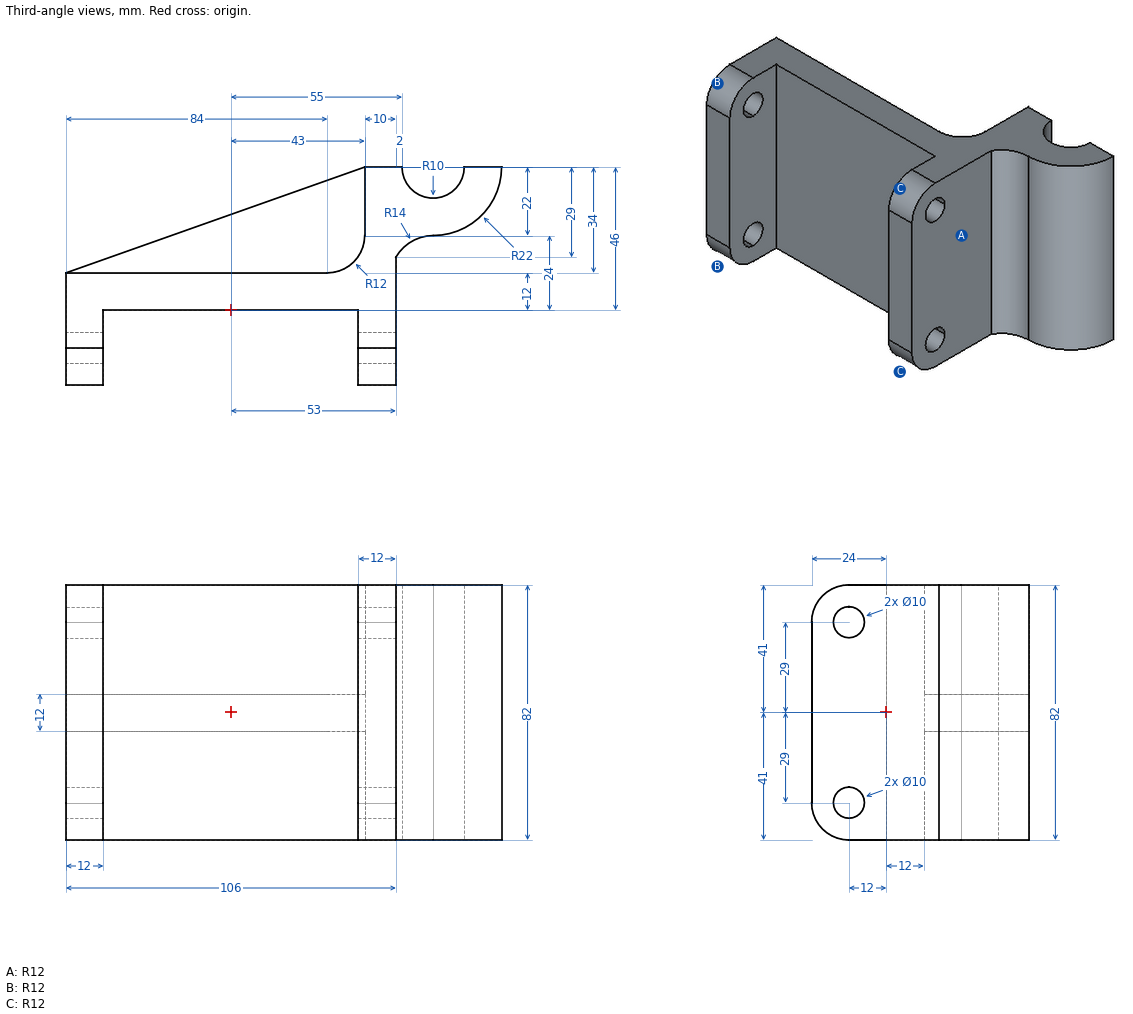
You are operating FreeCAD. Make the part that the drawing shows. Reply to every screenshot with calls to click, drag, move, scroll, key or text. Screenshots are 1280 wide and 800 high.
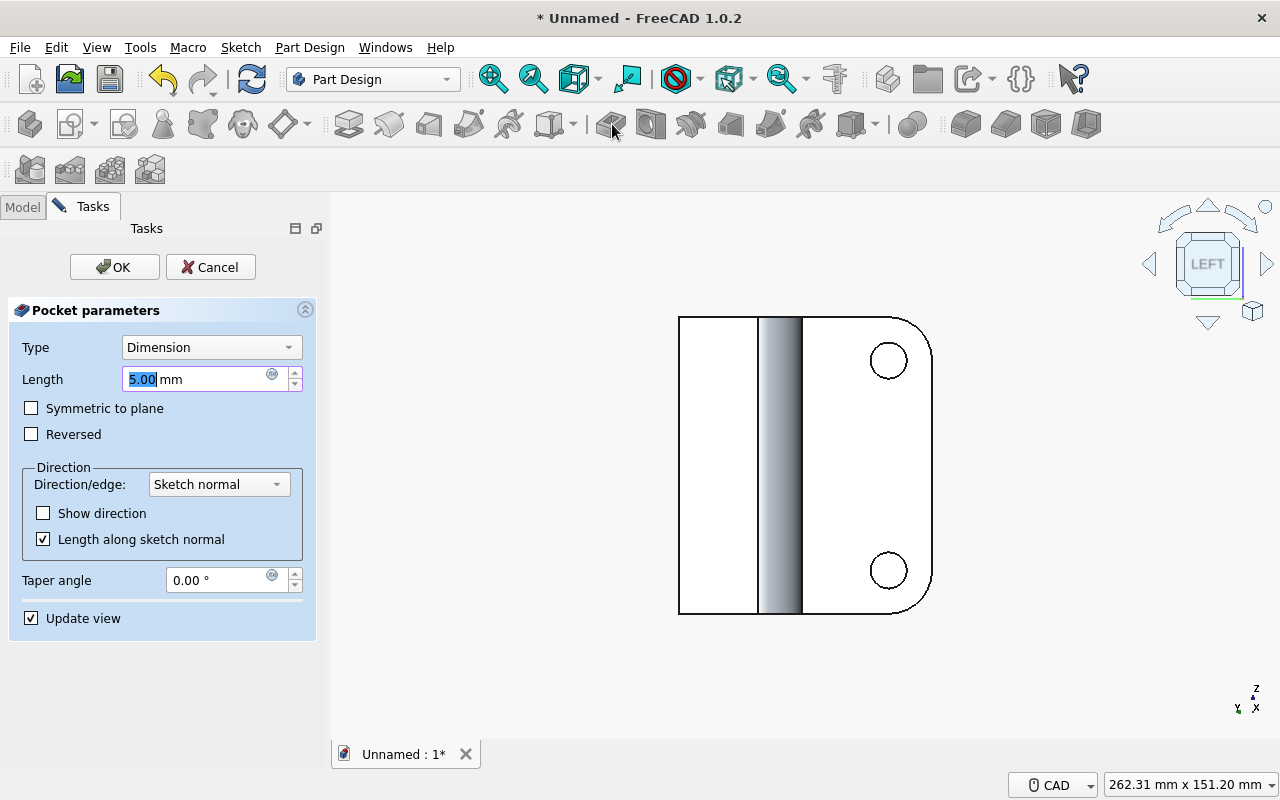
click(212, 348)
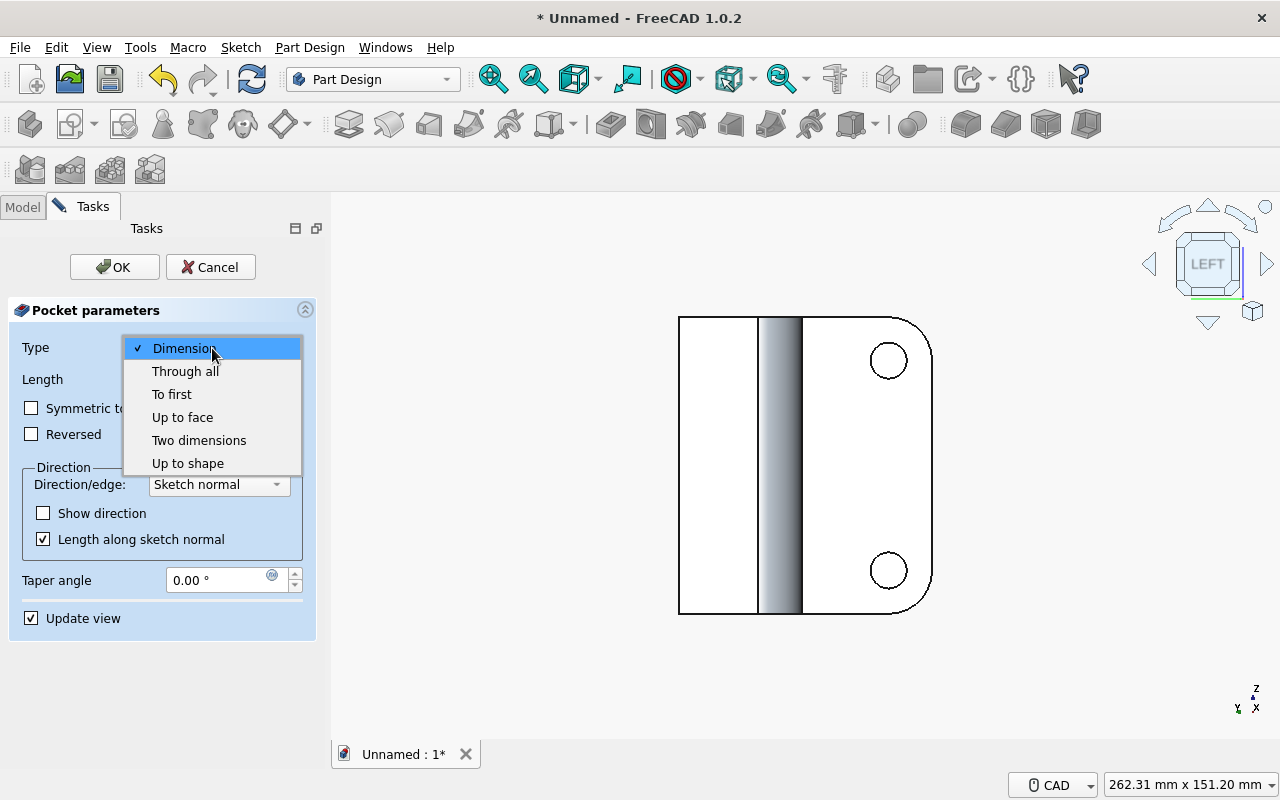
click(212, 372)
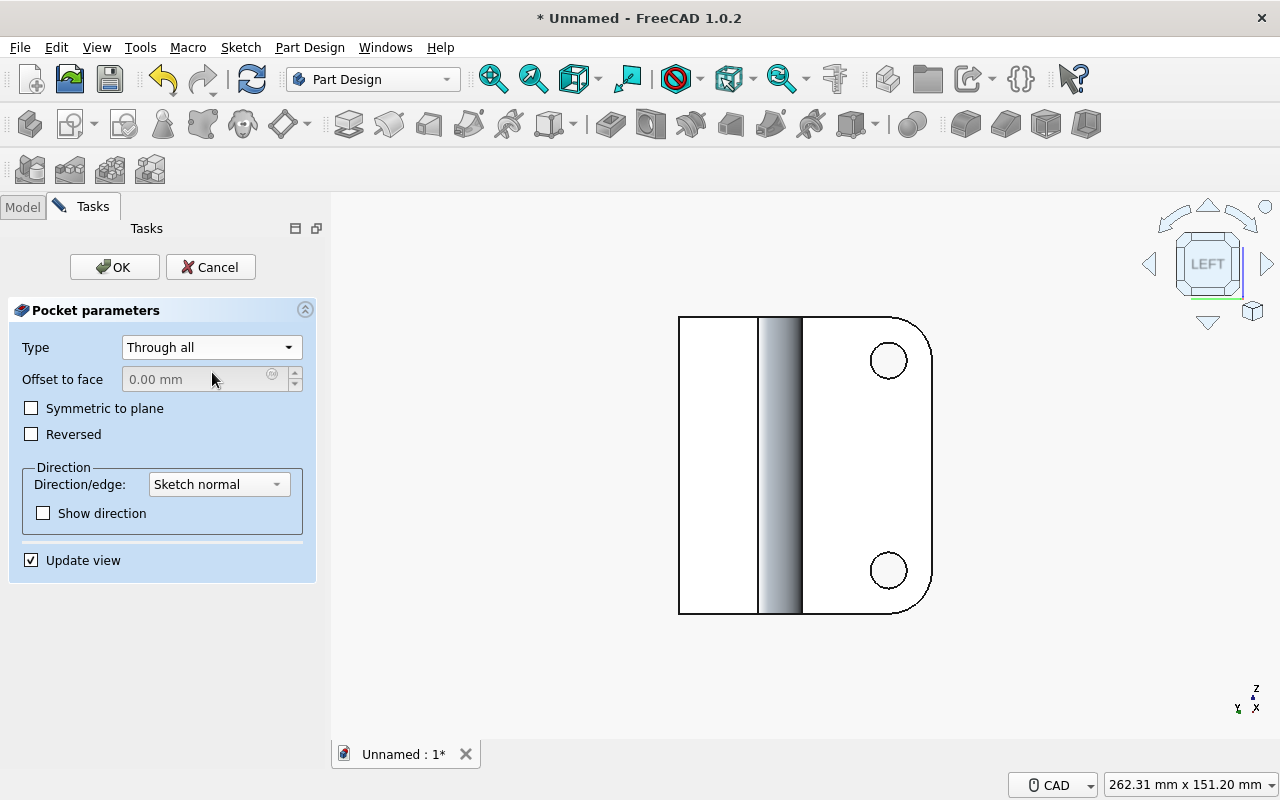
click(115, 267)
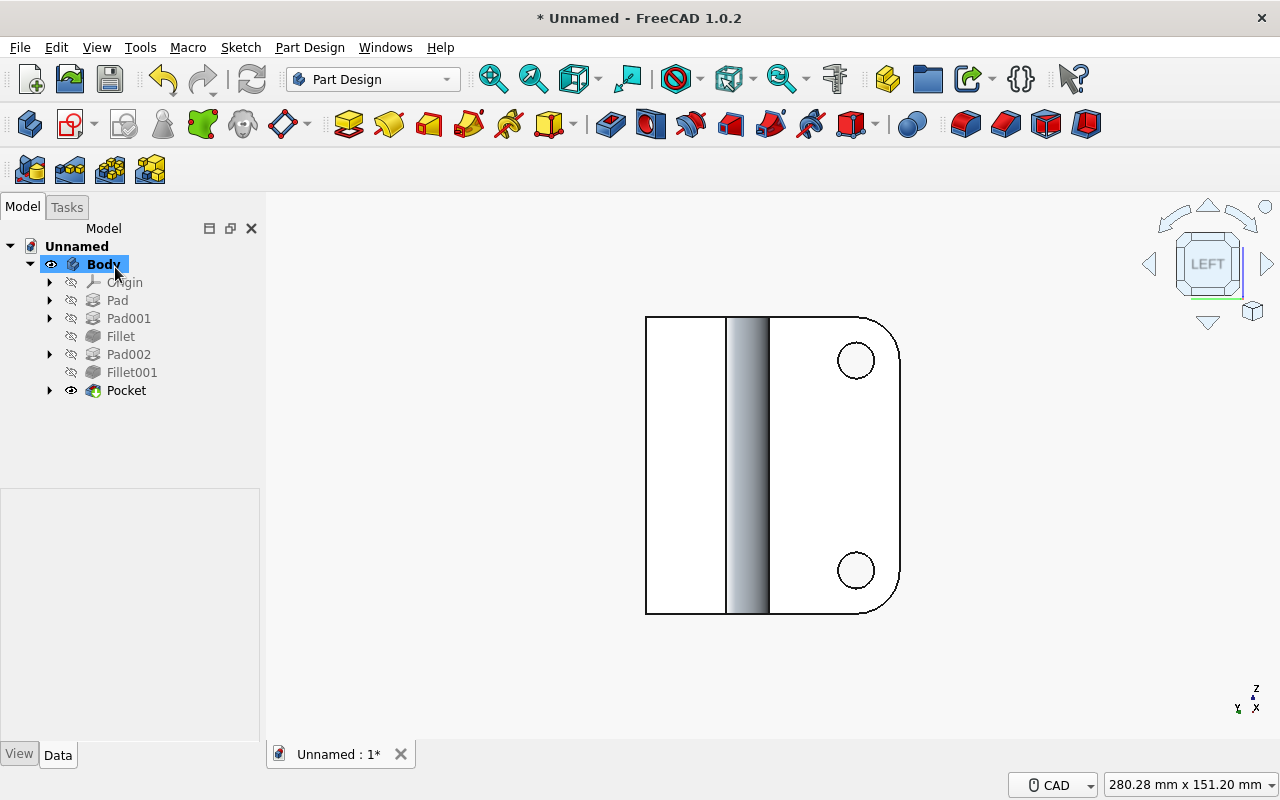
key(0)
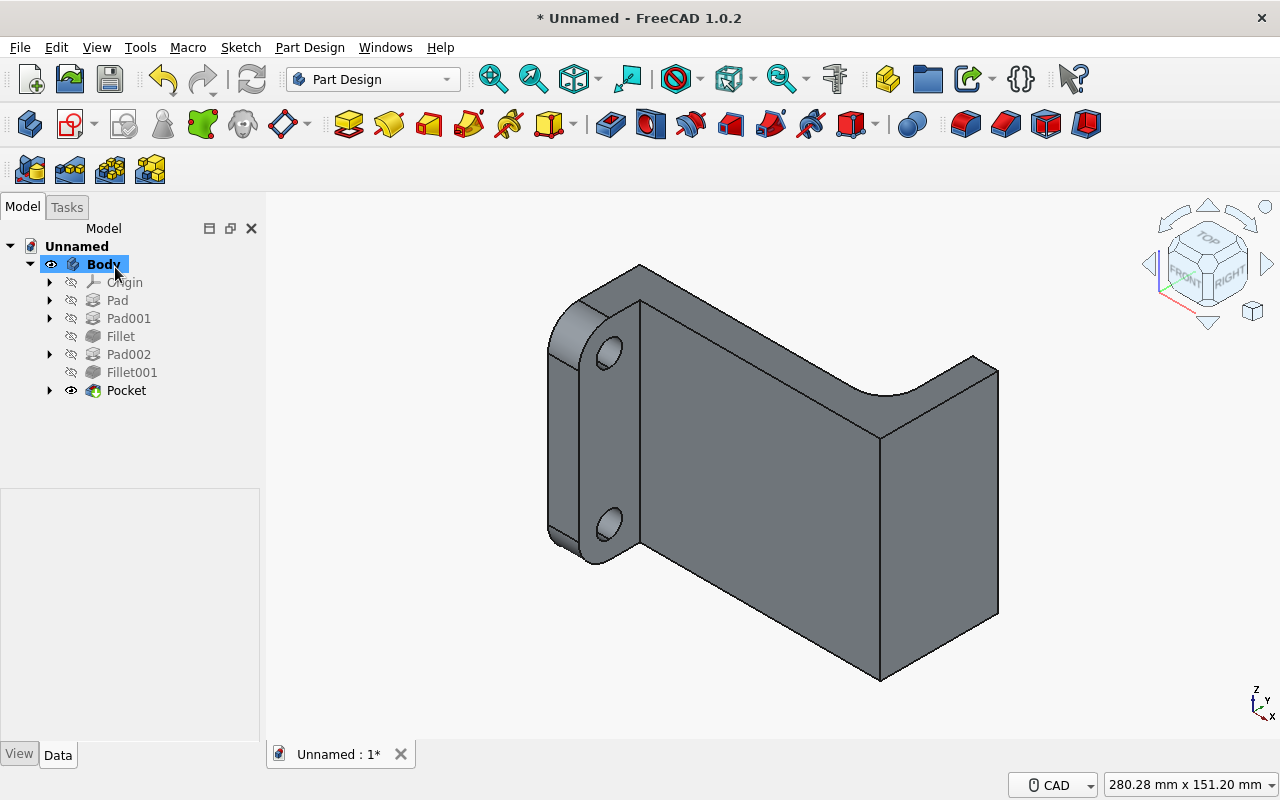
click(939, 560)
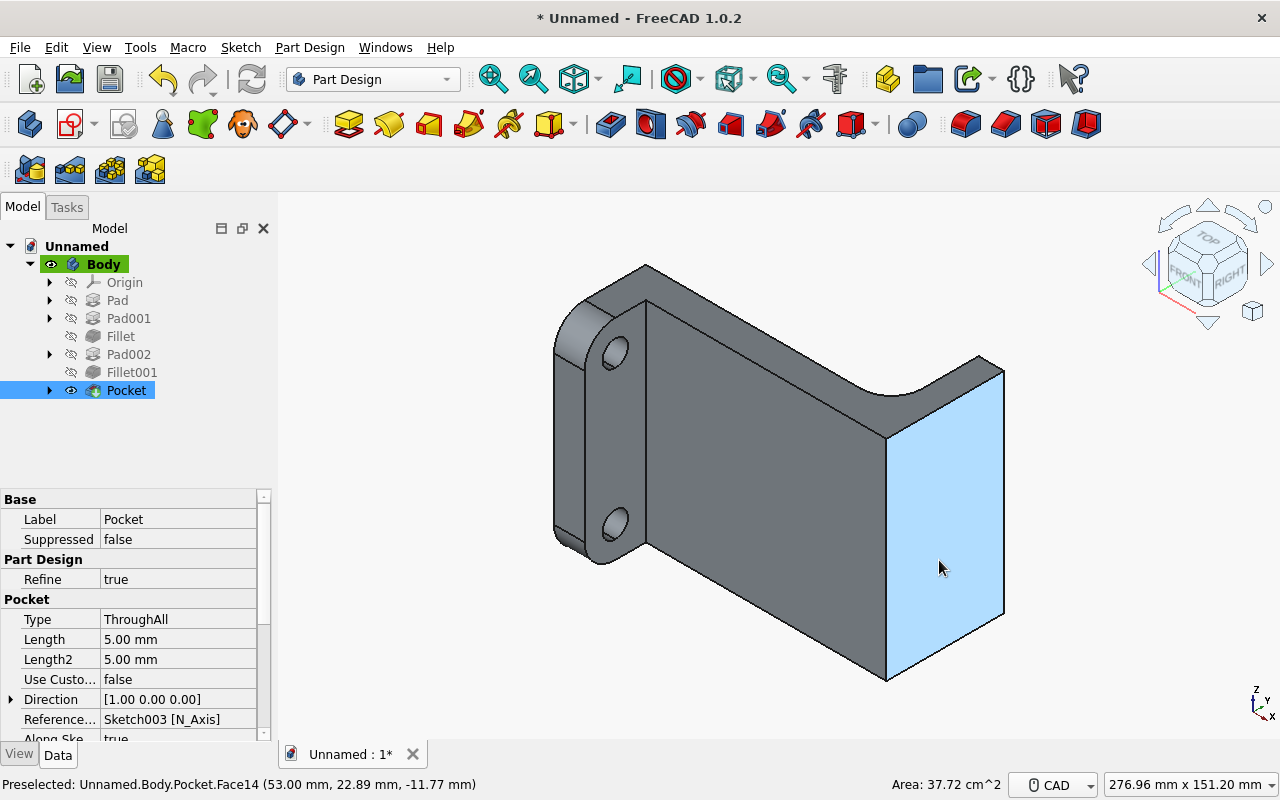
click(70, 124)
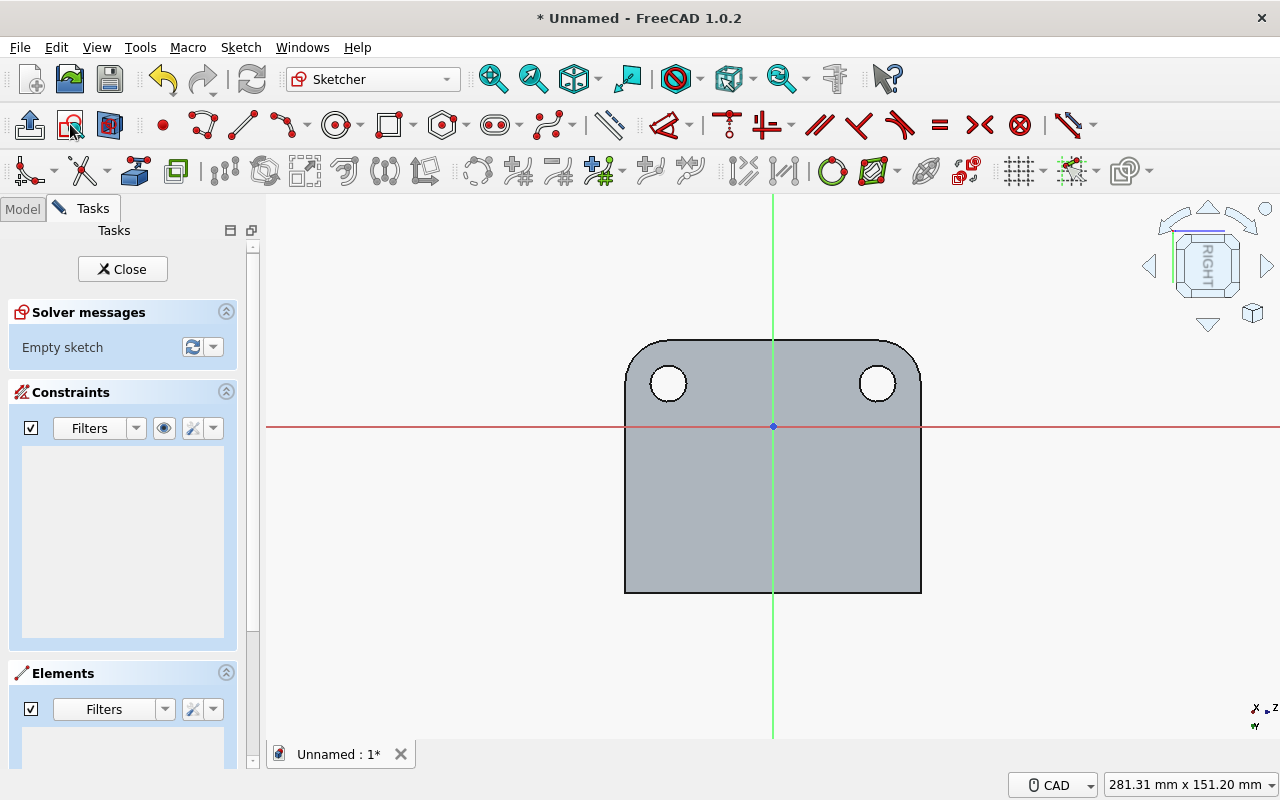
scroll(856, 283, up, 3)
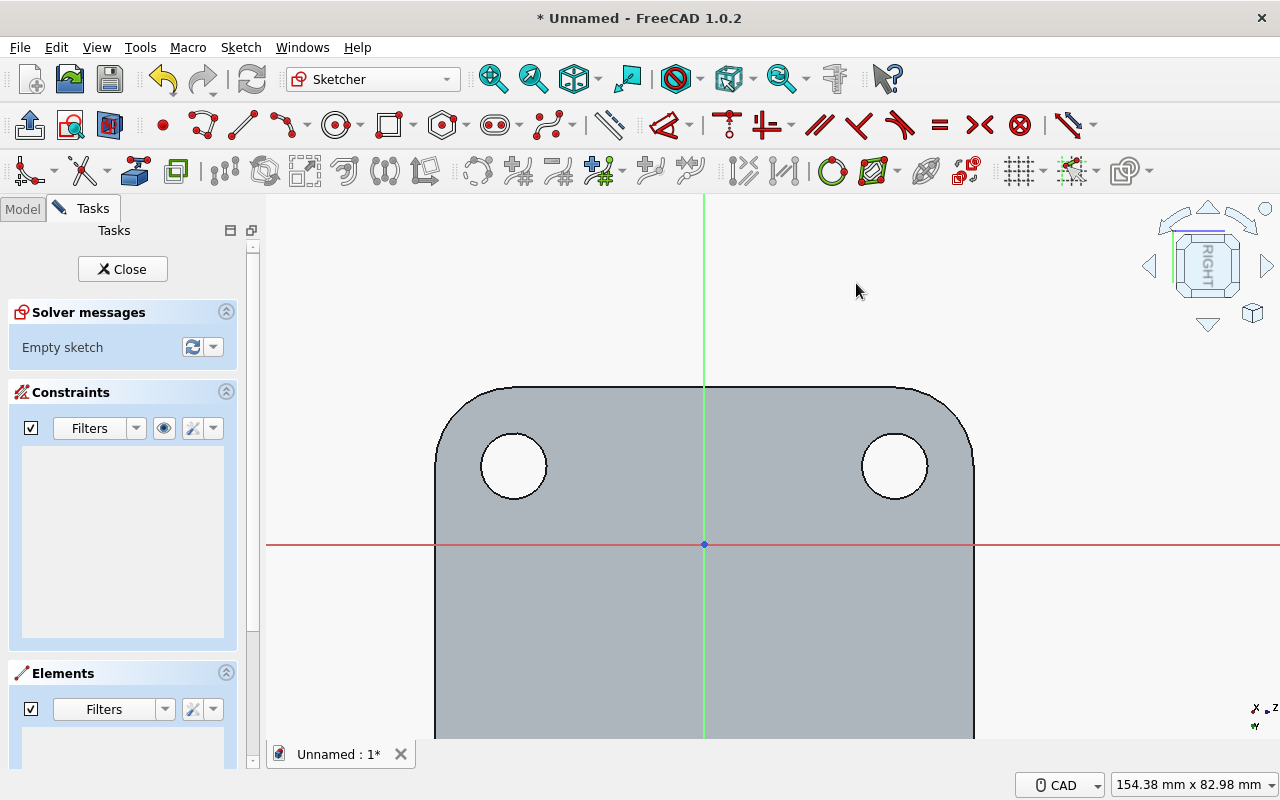
key(g)
key(r)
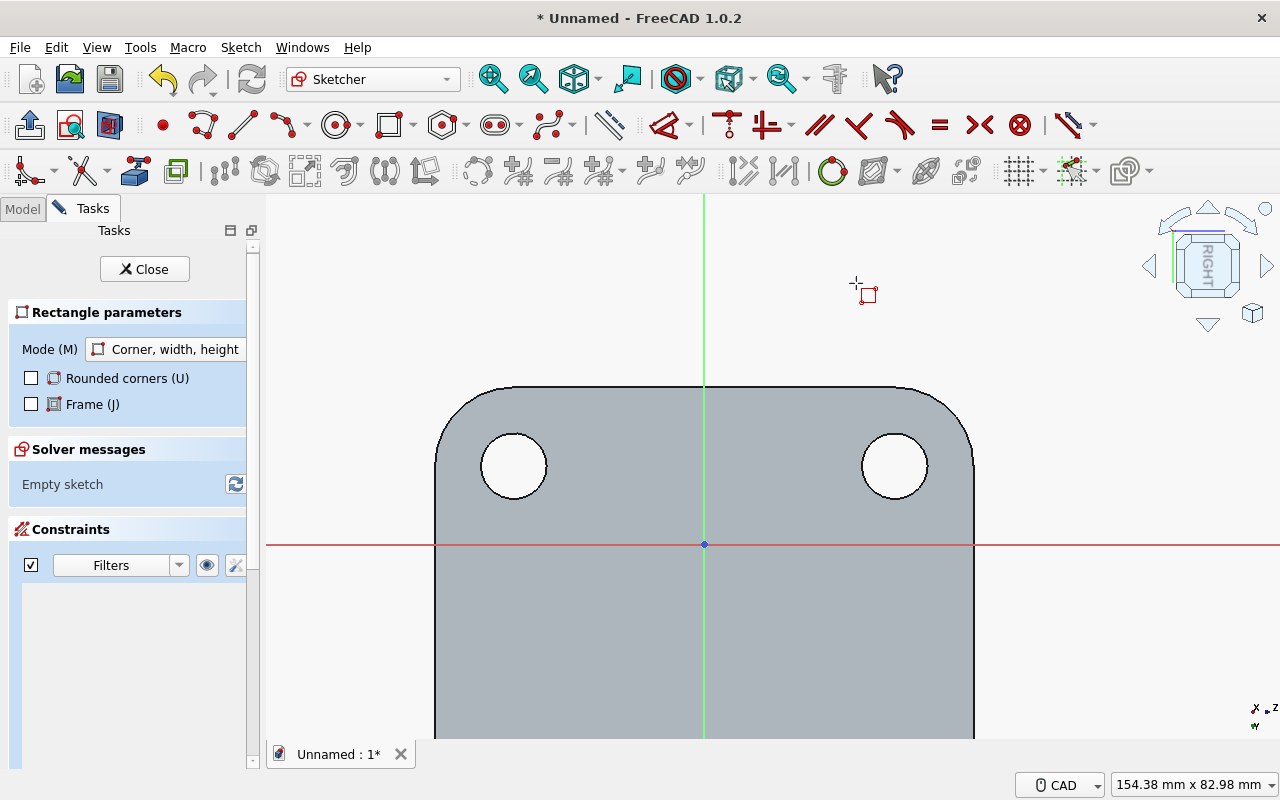
click(435, 387)
click(974, 545)
key(Escape)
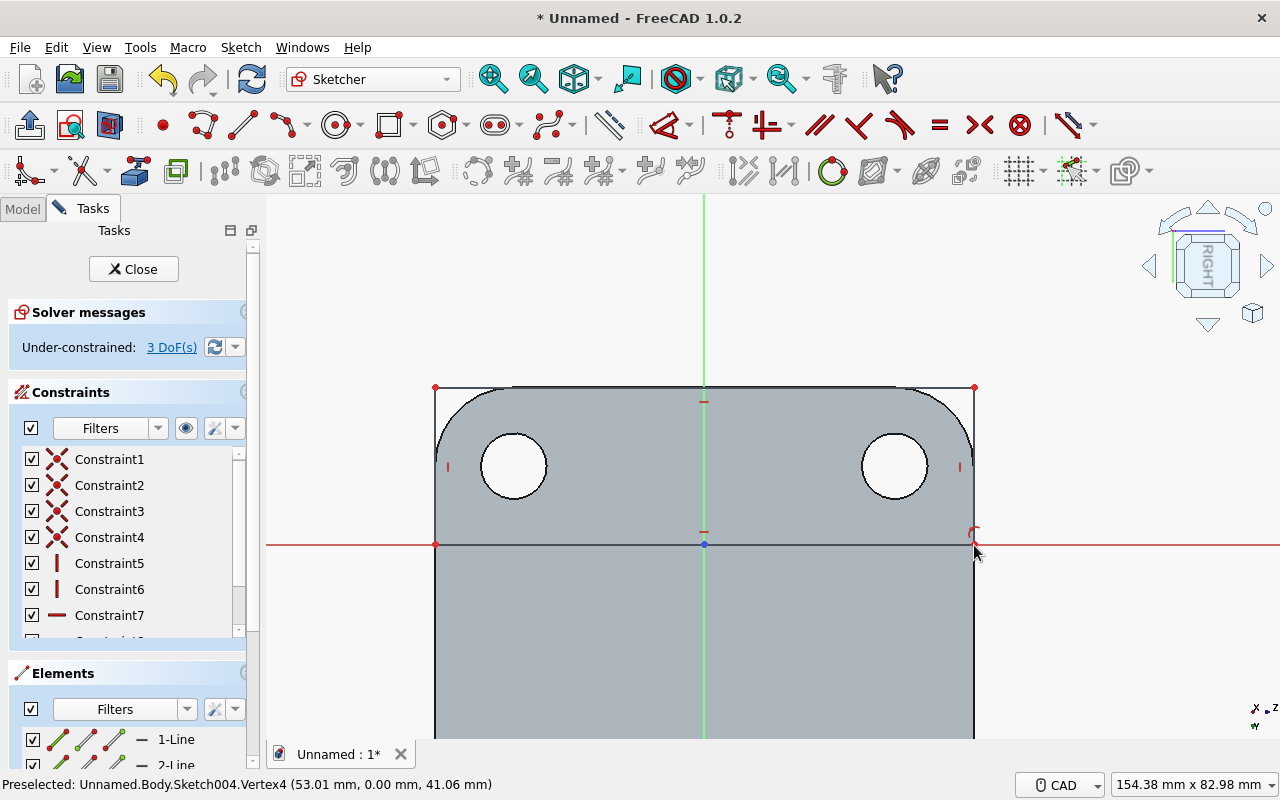
click(664, 126)